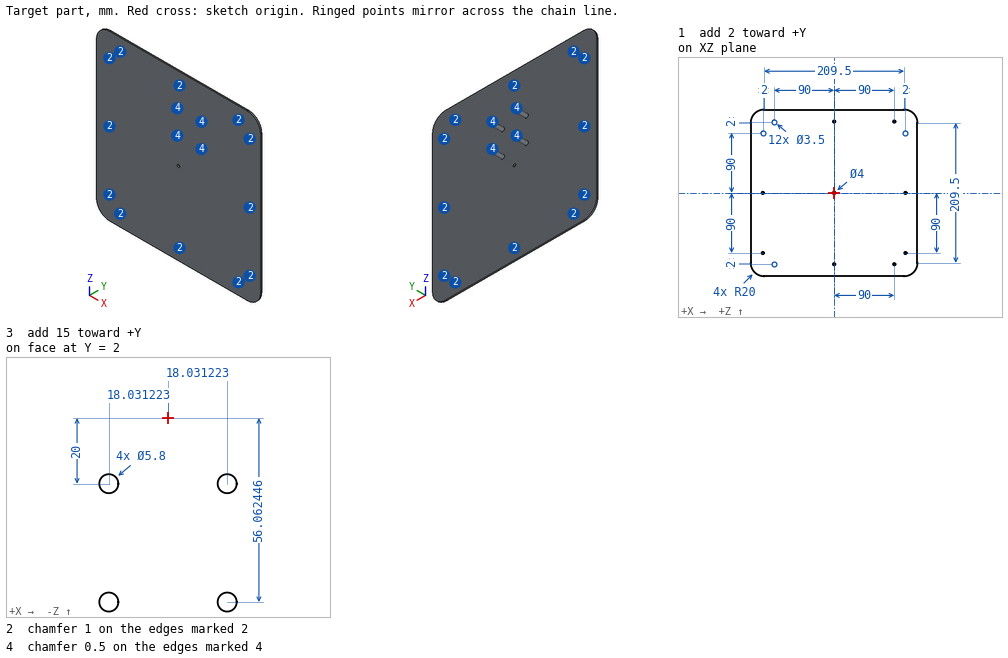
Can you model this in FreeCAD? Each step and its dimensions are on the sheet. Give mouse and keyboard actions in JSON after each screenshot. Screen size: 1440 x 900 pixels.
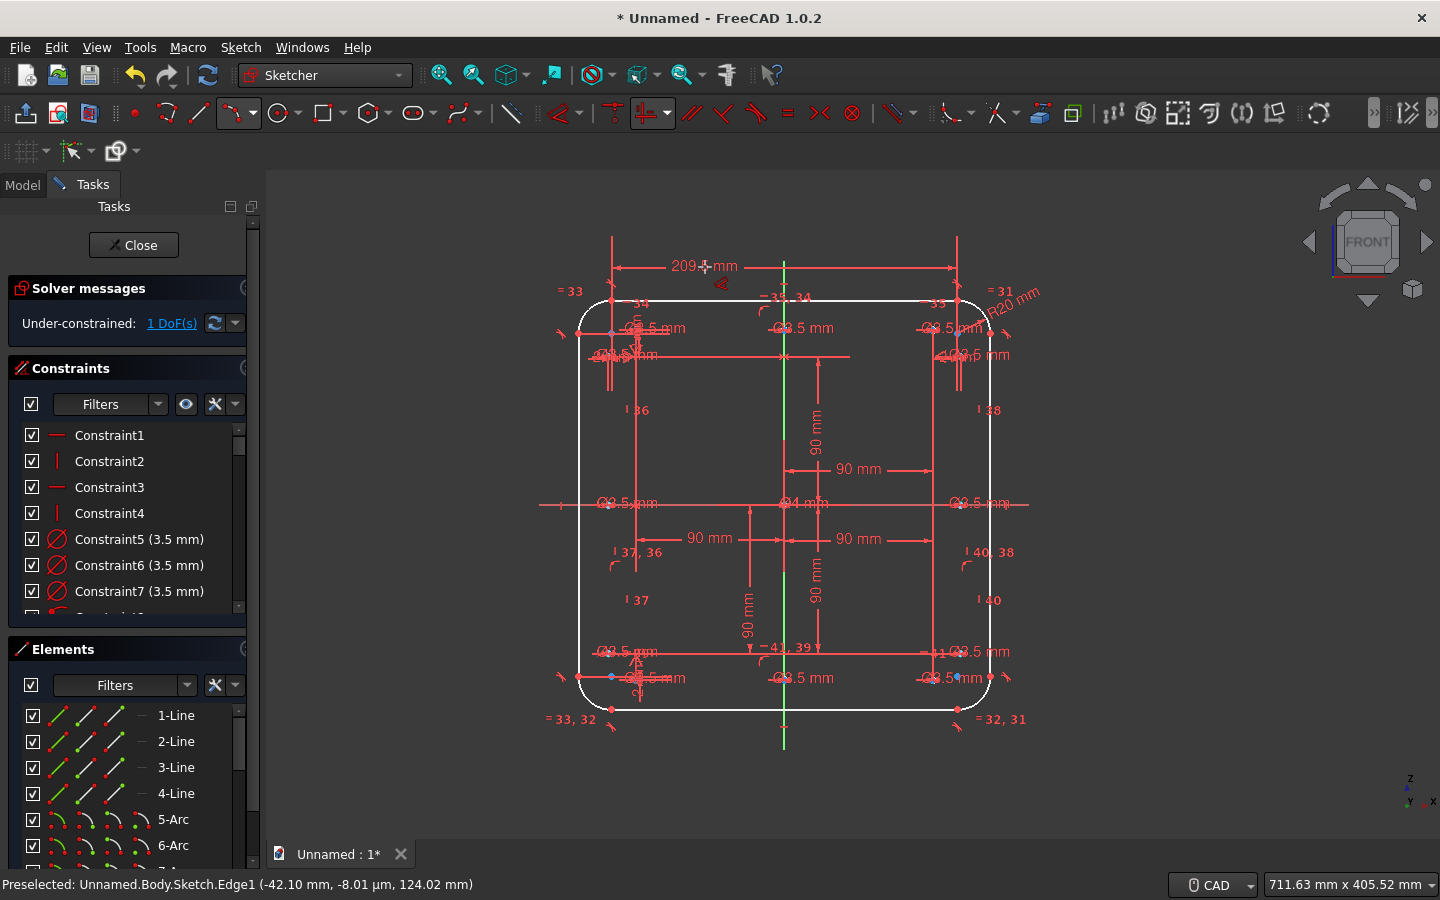
{"action": "left_click", "coordinate": [990, 437]}
{"action": "left_click", "coordinate": [1024, 426]}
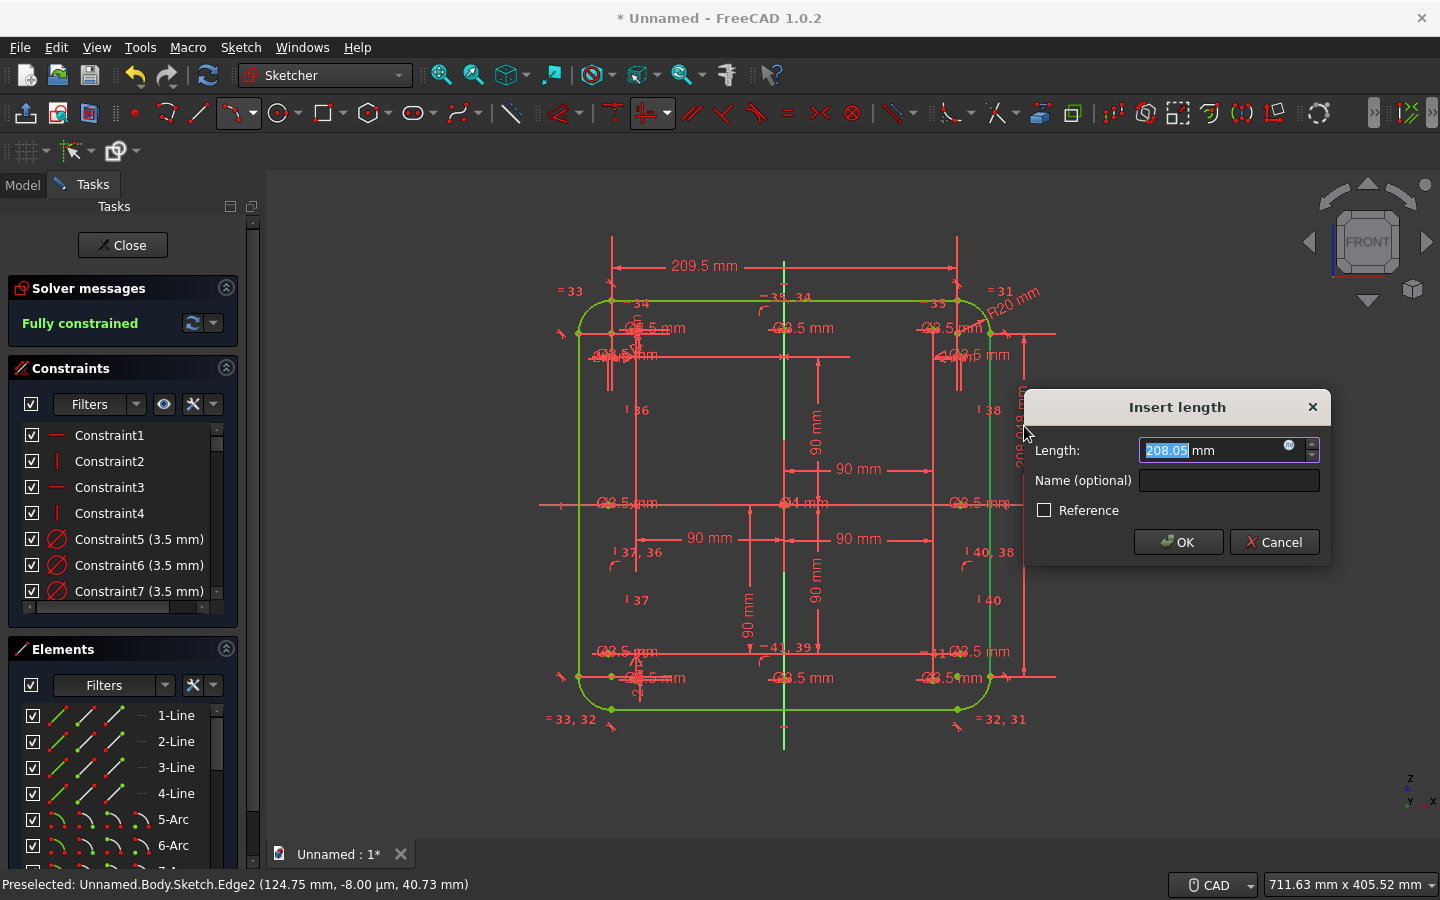
{"action": "type", "text": "209.5"}
{"action": "key", "text": "Return"}
{"action": "key", "text": "Escape"}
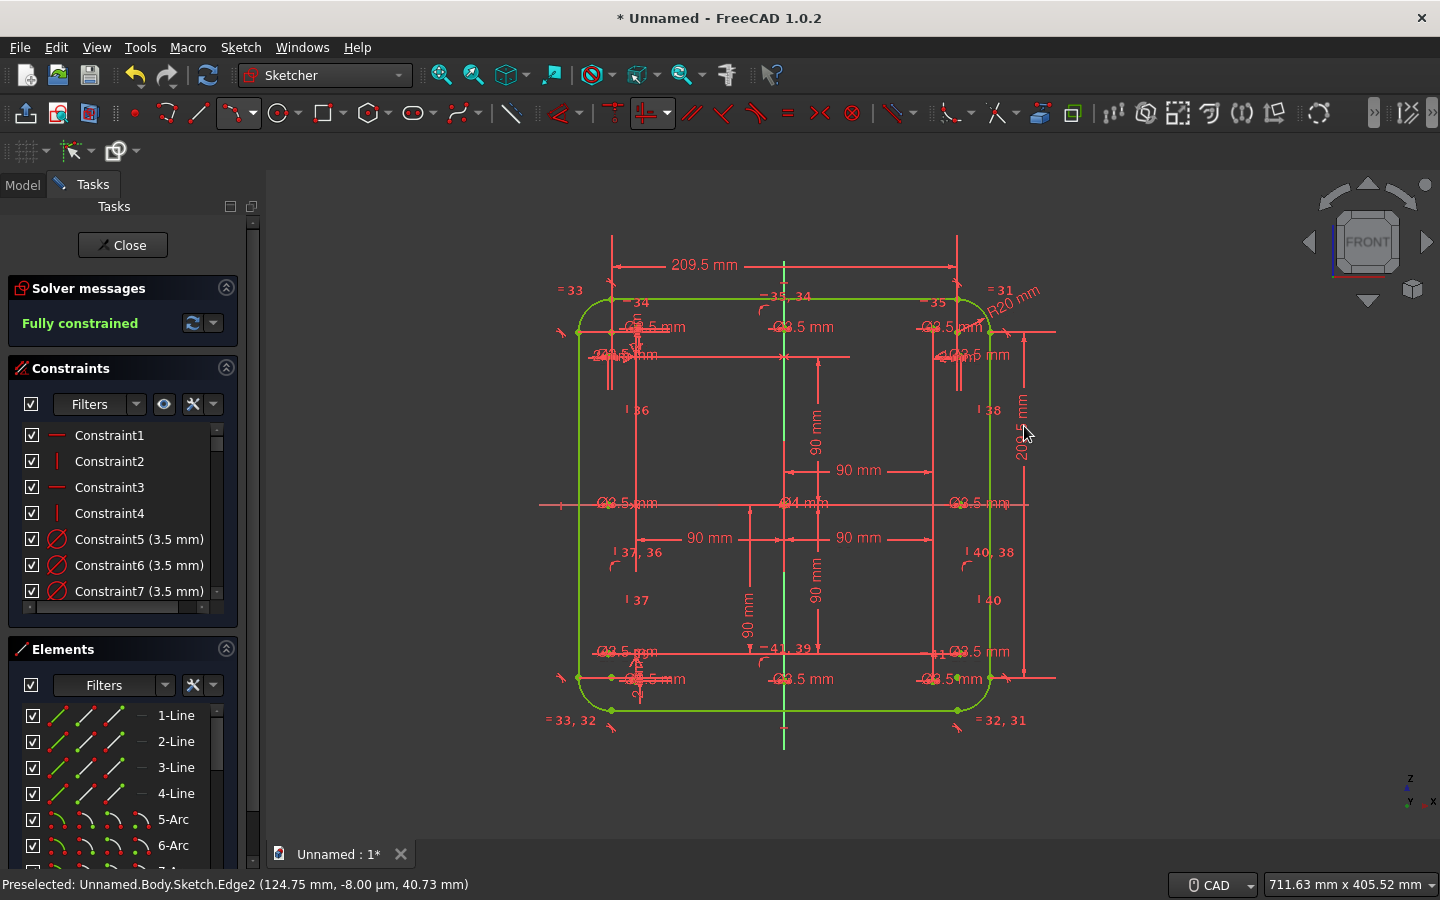
{"action": "left_click", "coordinate": [123, 245]}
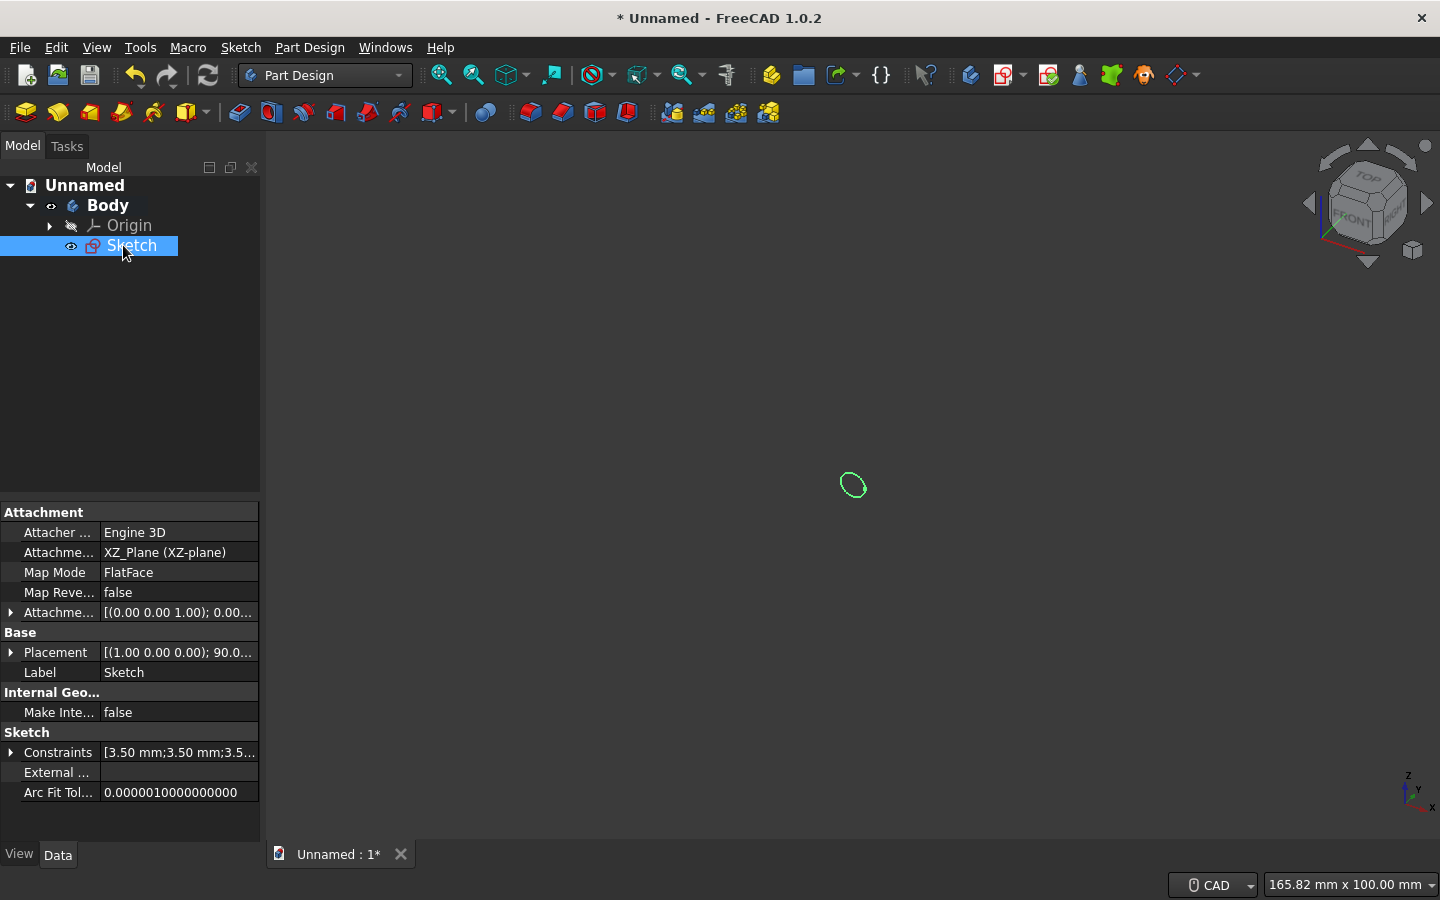
{"action": "left_click", "coordinate": [26, 112]}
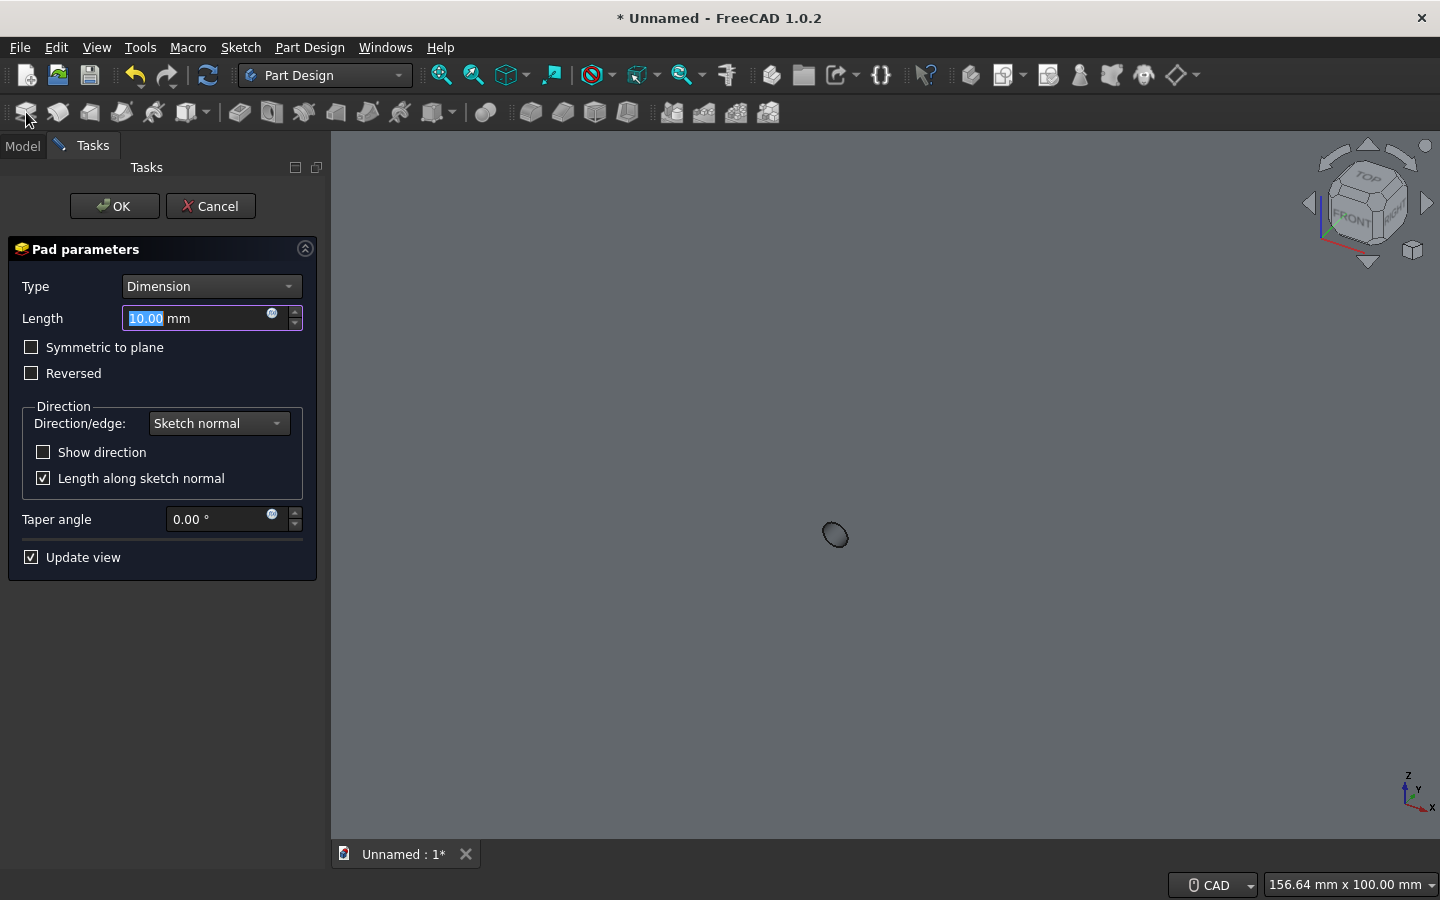
{"action": "type", "text": "2"}
{"action": "key", "text": "Tab"}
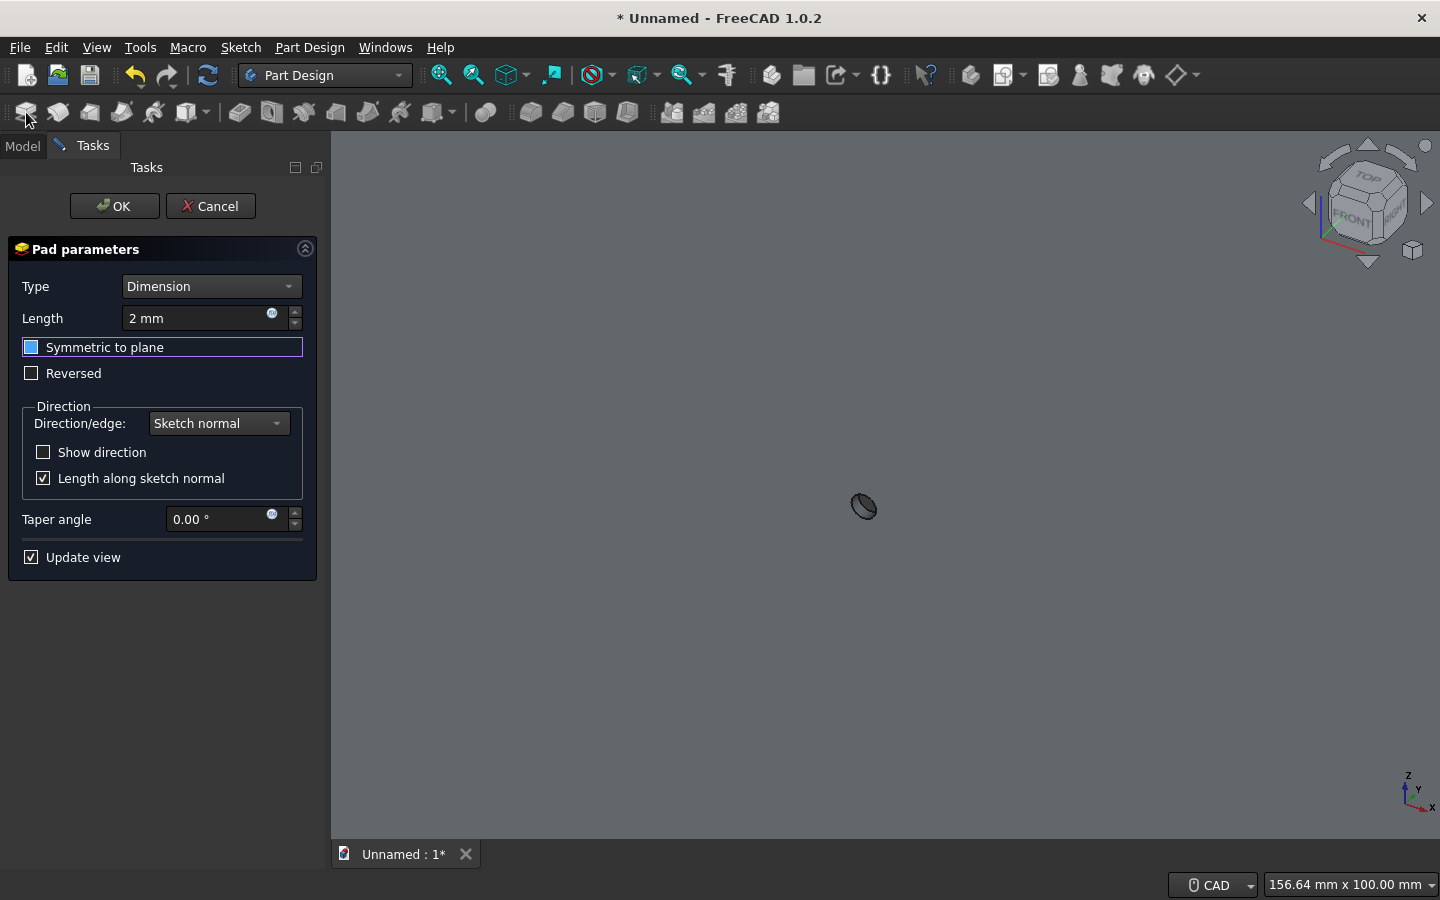
{"action": "left_click", "coordinate": [30, 373]}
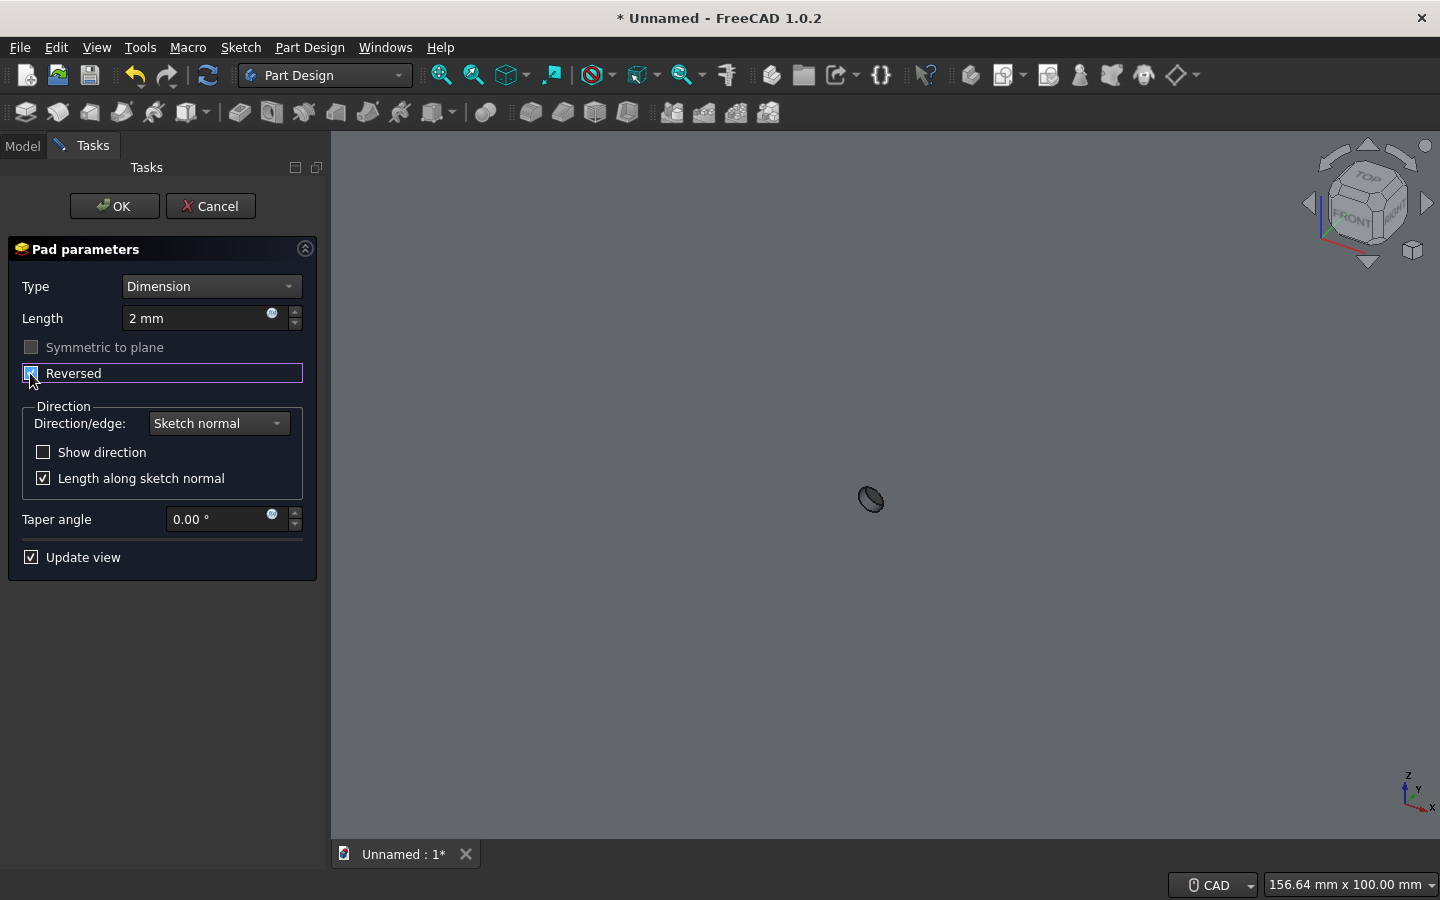
{"action": "left_click", "coordinate": [115, 206]}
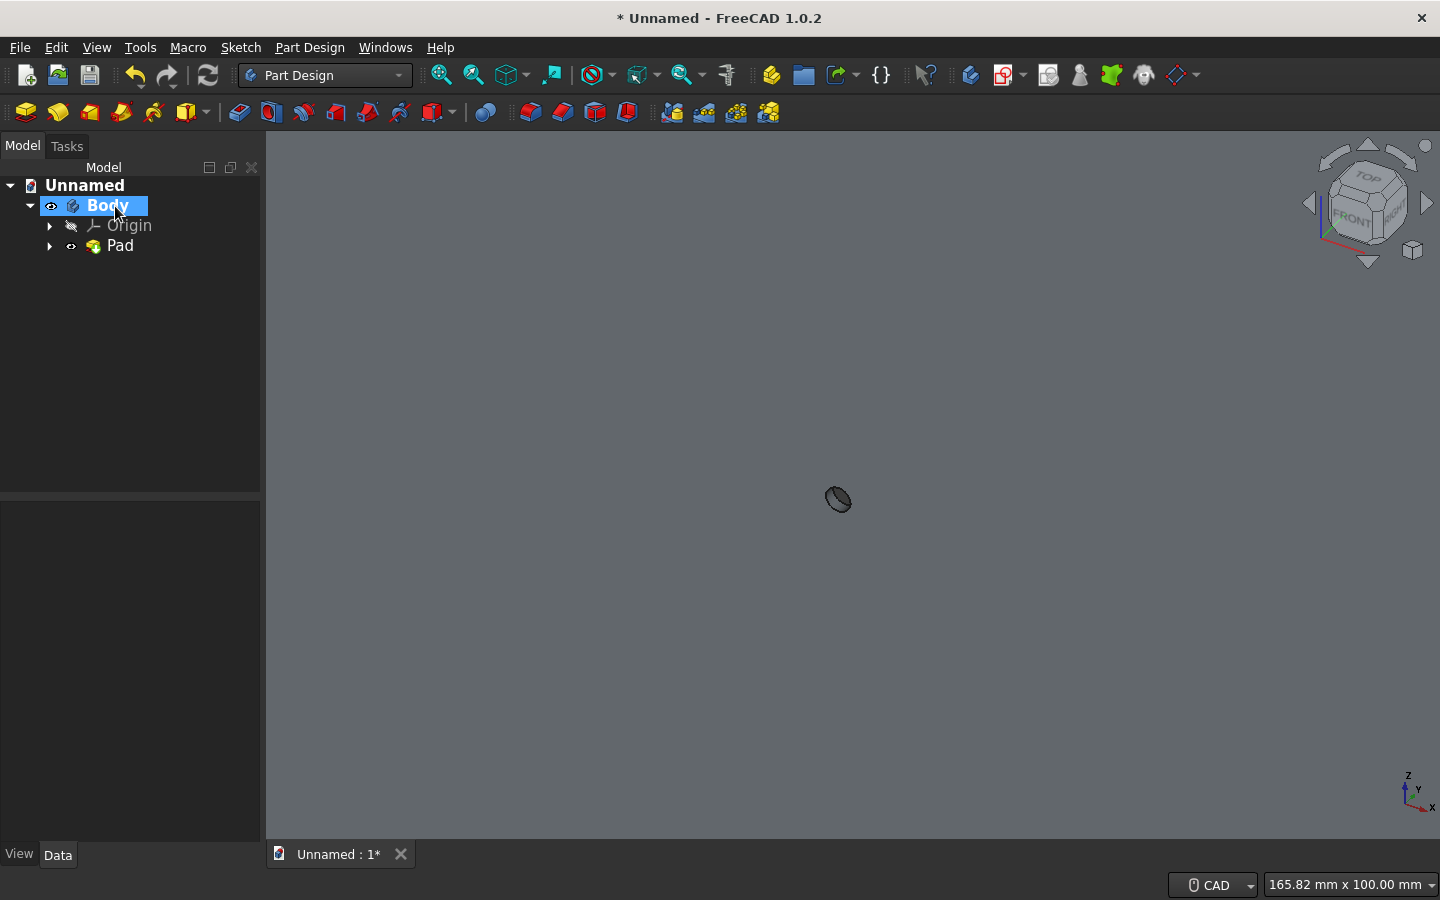
{"action": "key", "text": "v f"}